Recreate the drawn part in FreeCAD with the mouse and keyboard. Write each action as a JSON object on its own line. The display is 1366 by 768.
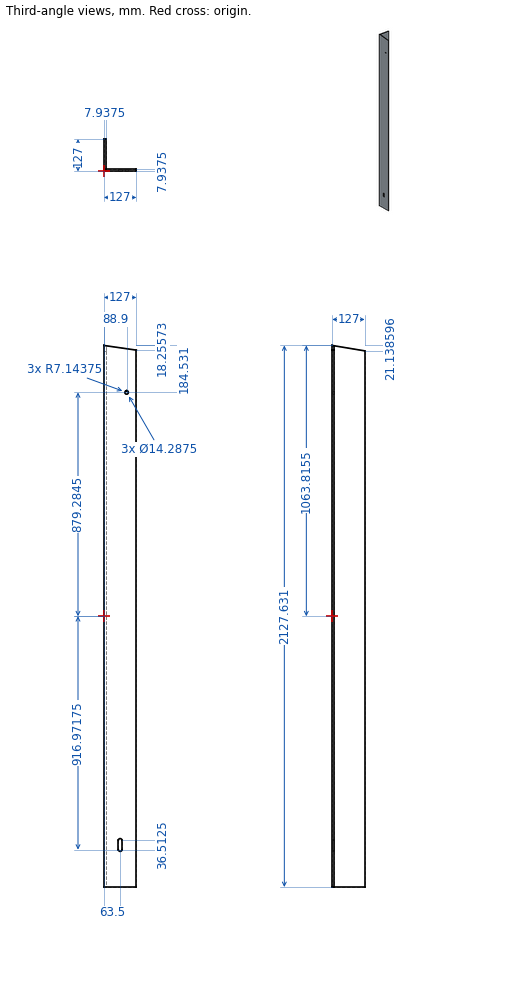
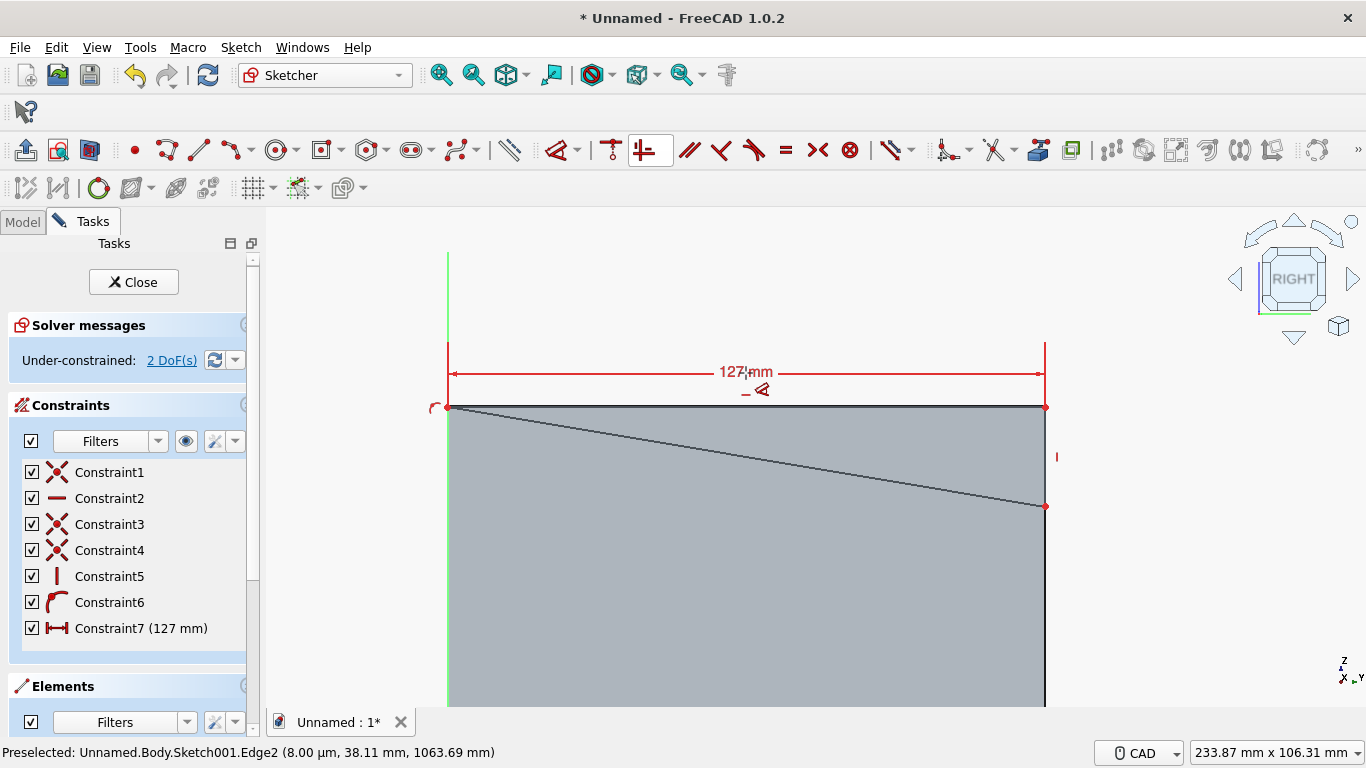
{"action": "left_click", "coordinate": [1045, 437]}
{"action": "left_click", "coordinate": [1079, 457]}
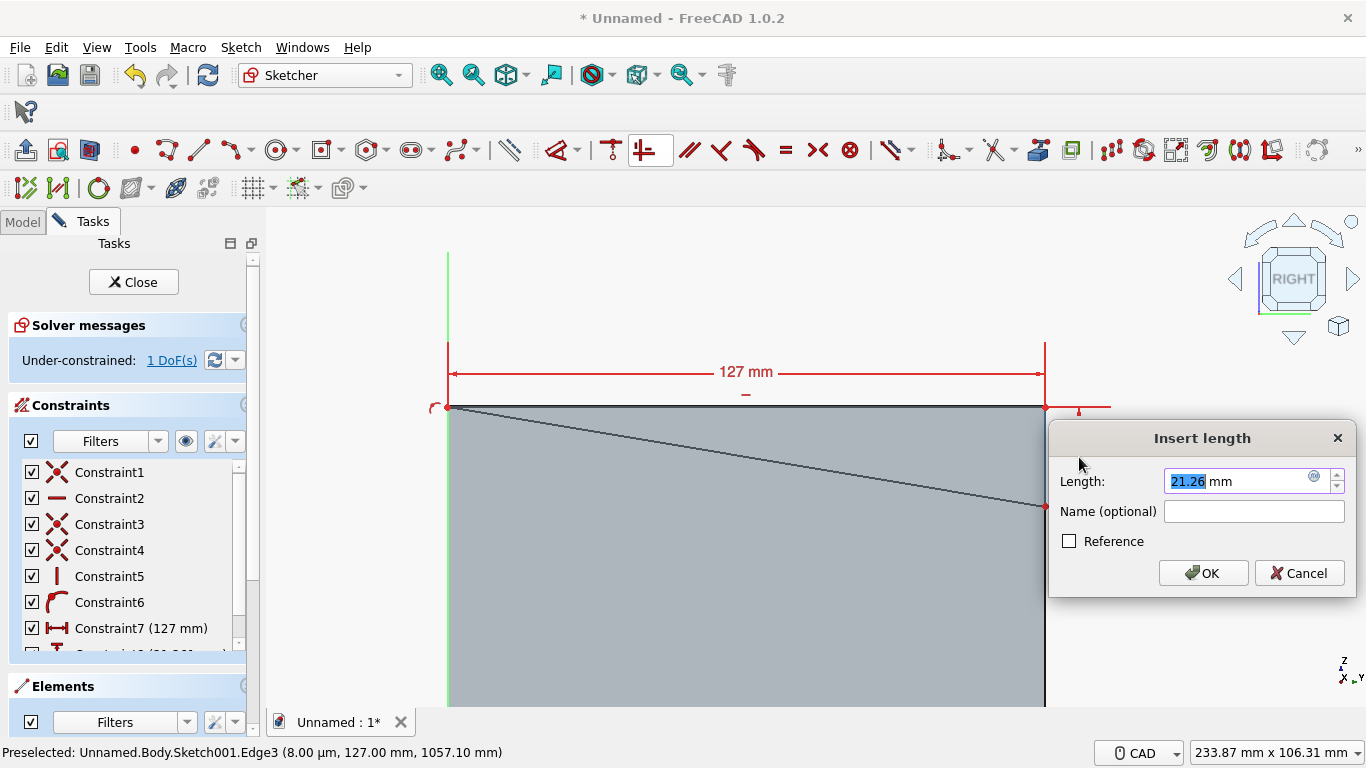
{"action": "type", "text": "21.138596"}
{"action": "key", "text": "Return"}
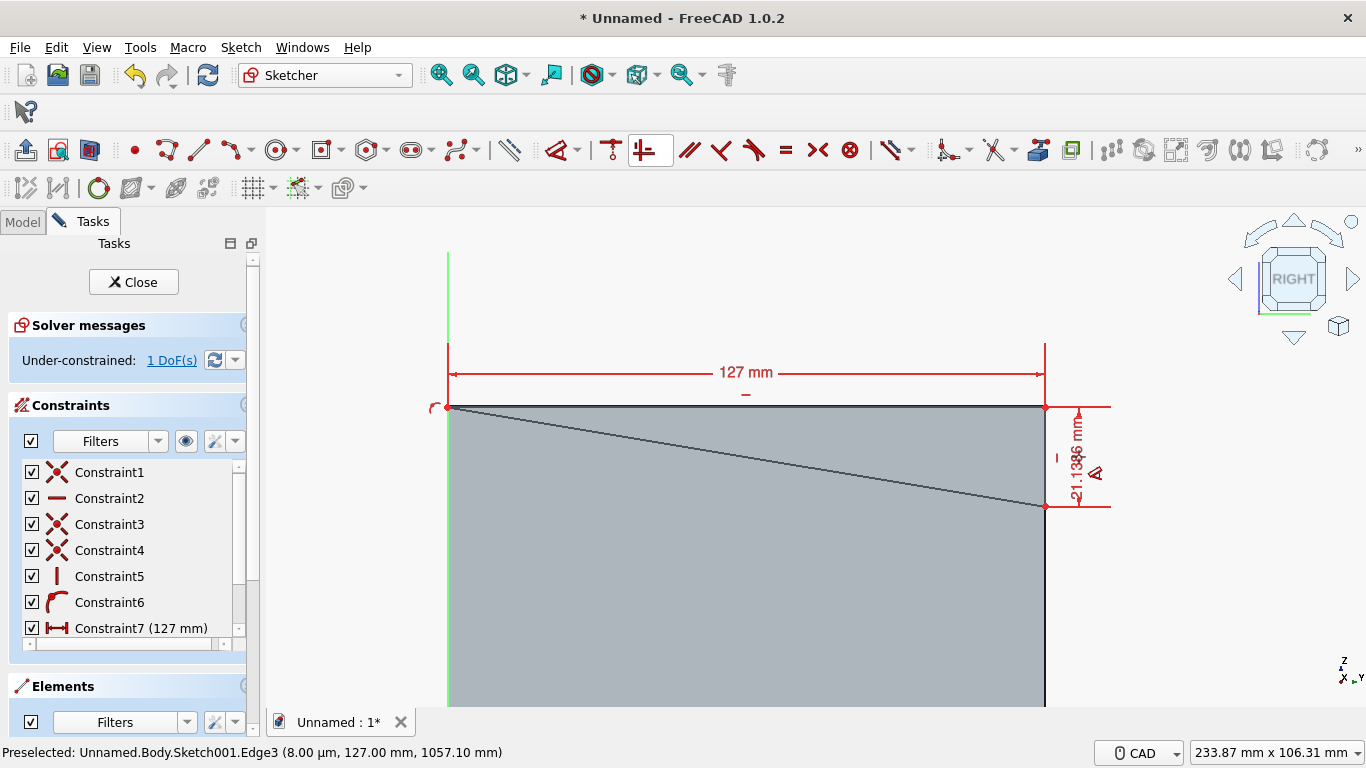
{"action": "left_click", "coordinate": [448, 407]}
{"action": "left_click", "coordinate": [414, 543]}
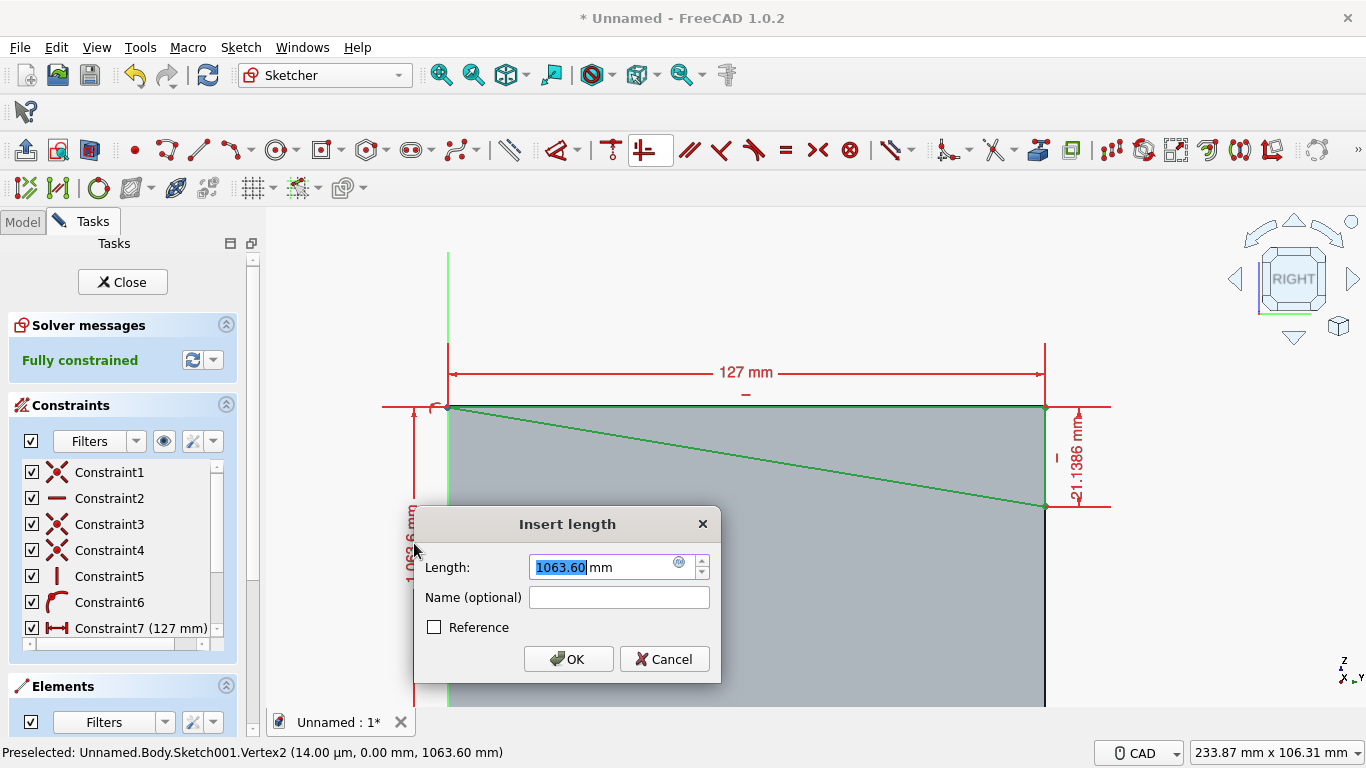
{"action": "type", "text": "1063.8155"}
{"action": "key", "text": "Return"}
{"action": "key", "text": "Escape"}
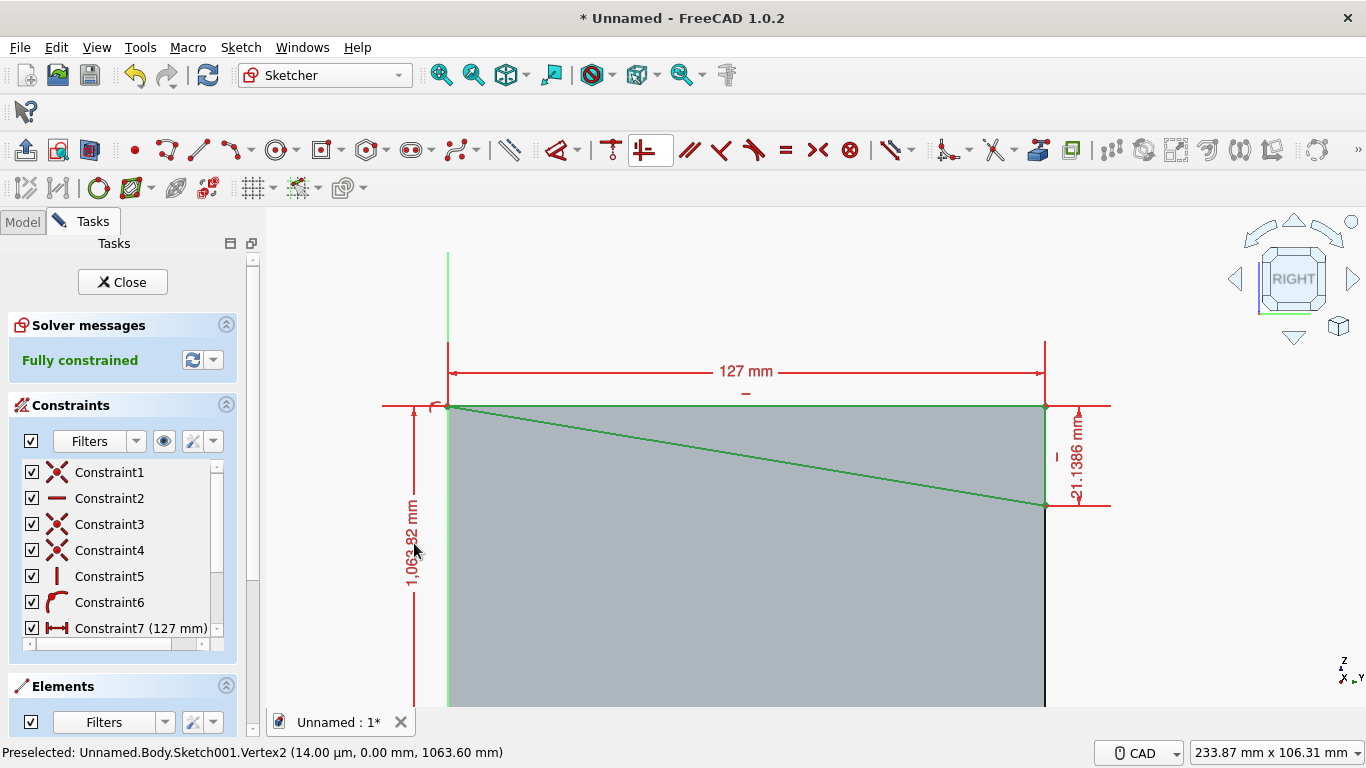
{"action": "left_click", "coordinate": [123, 282]}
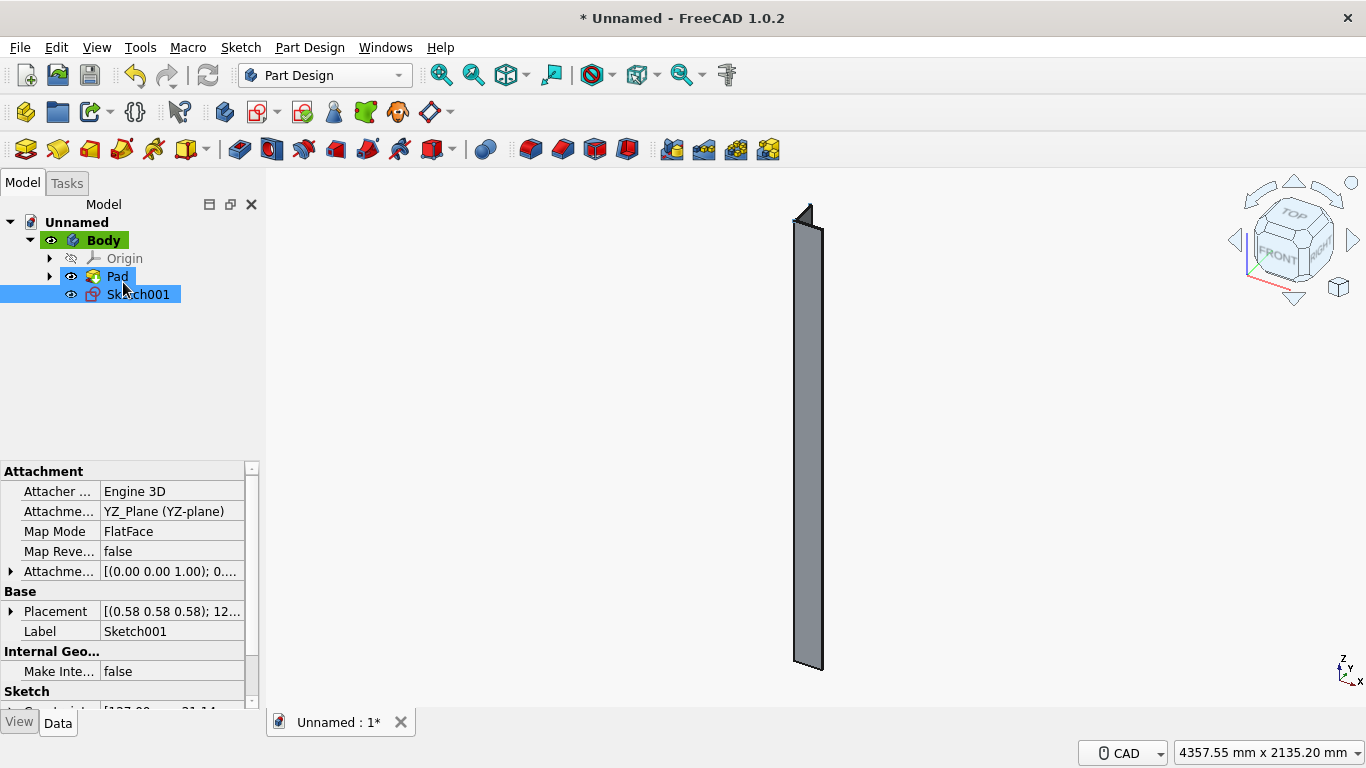
{"action": "left_click", "coordinate": [240, 150]}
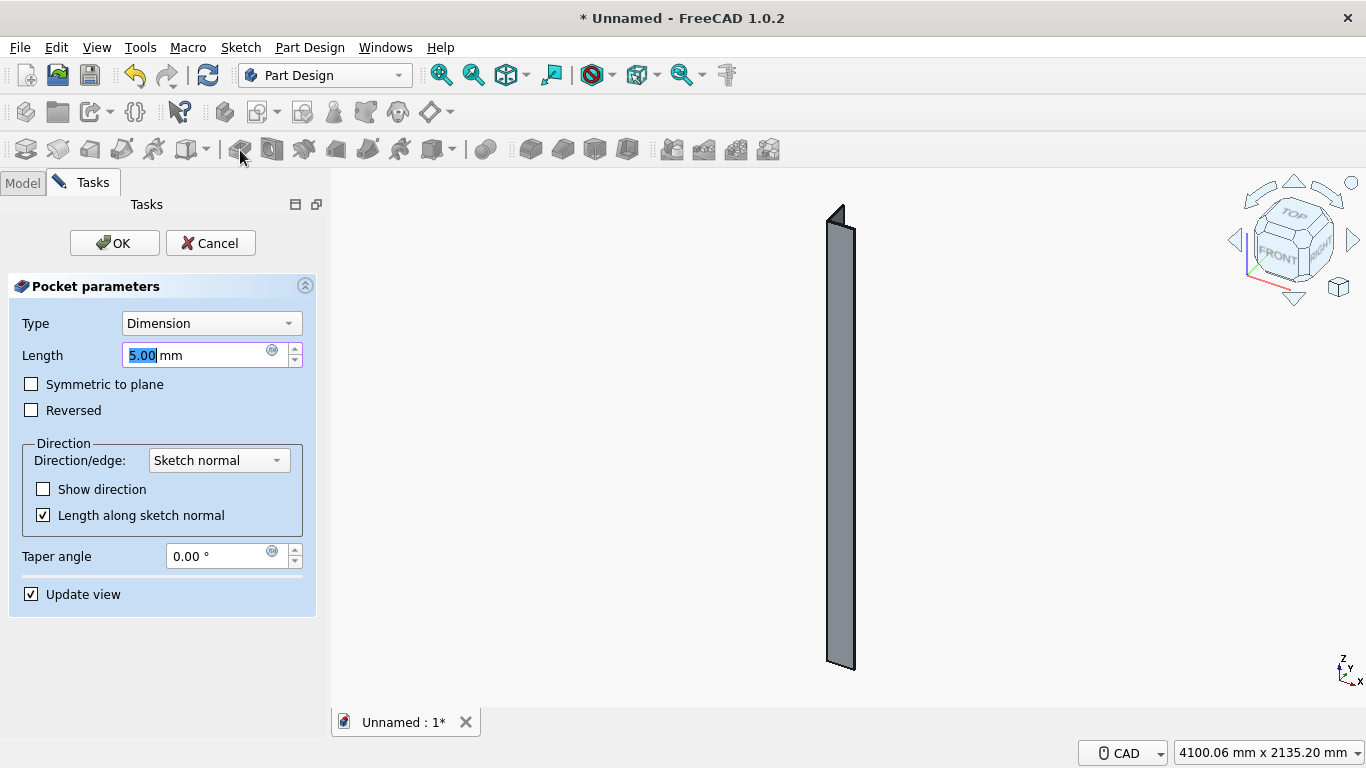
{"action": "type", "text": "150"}
{"action": "key", "text": "Tab"}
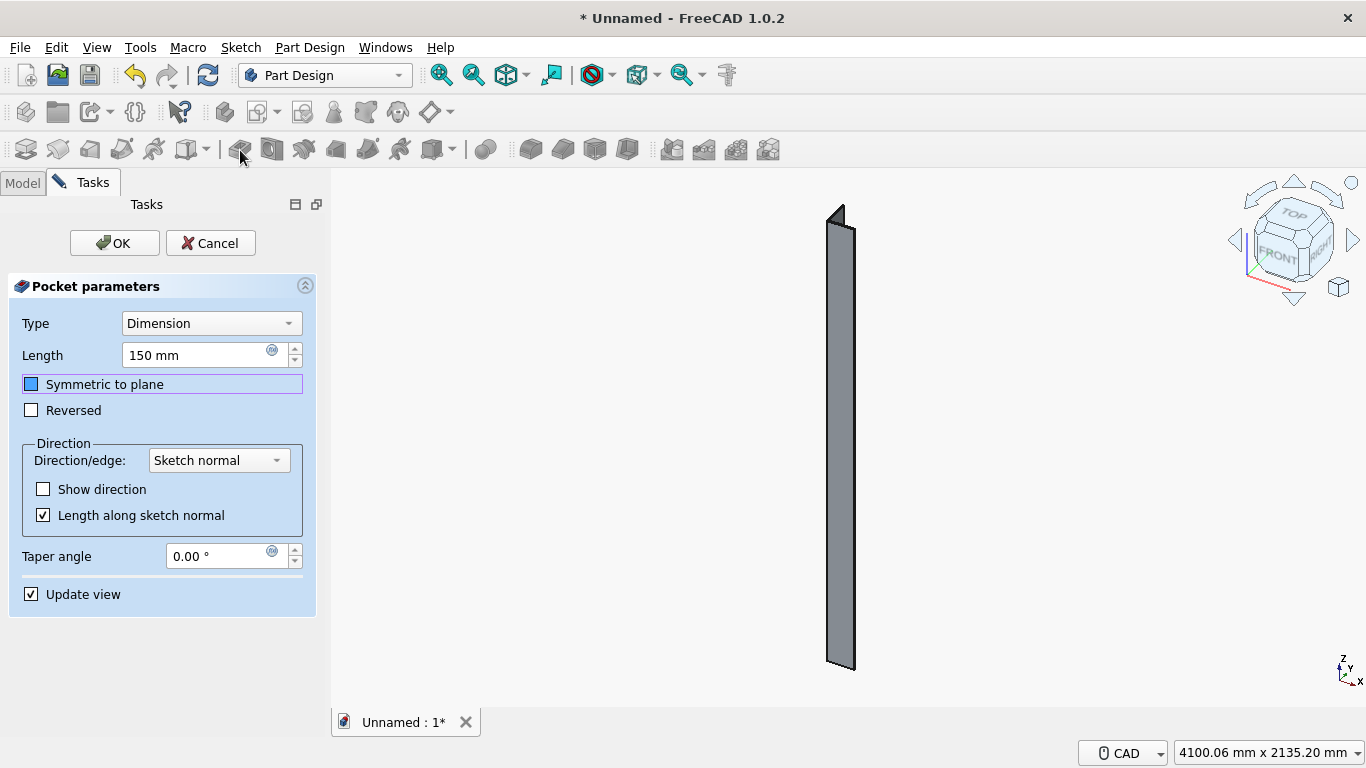
{"action": "left_click", "coordinate": [30, 410]}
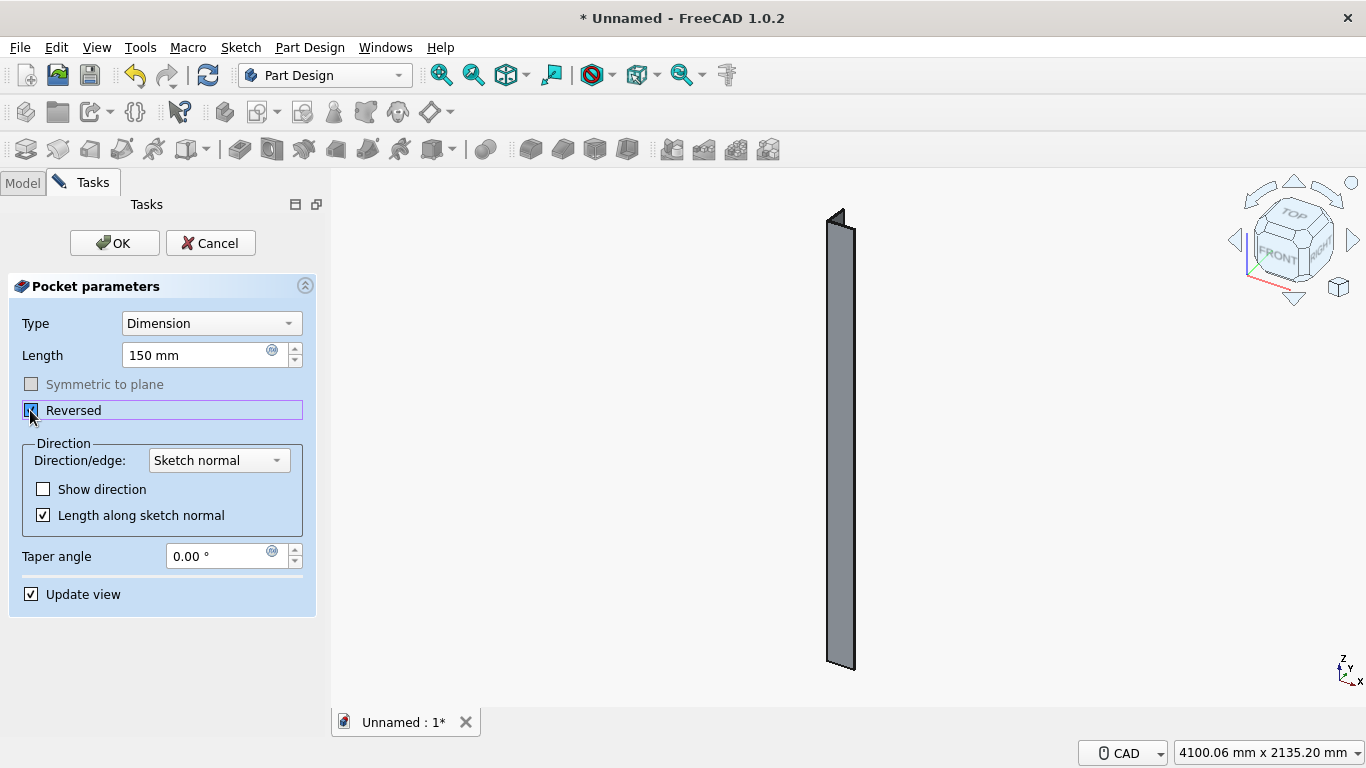
{"action": "left_click", "coordinate": [115, 243]}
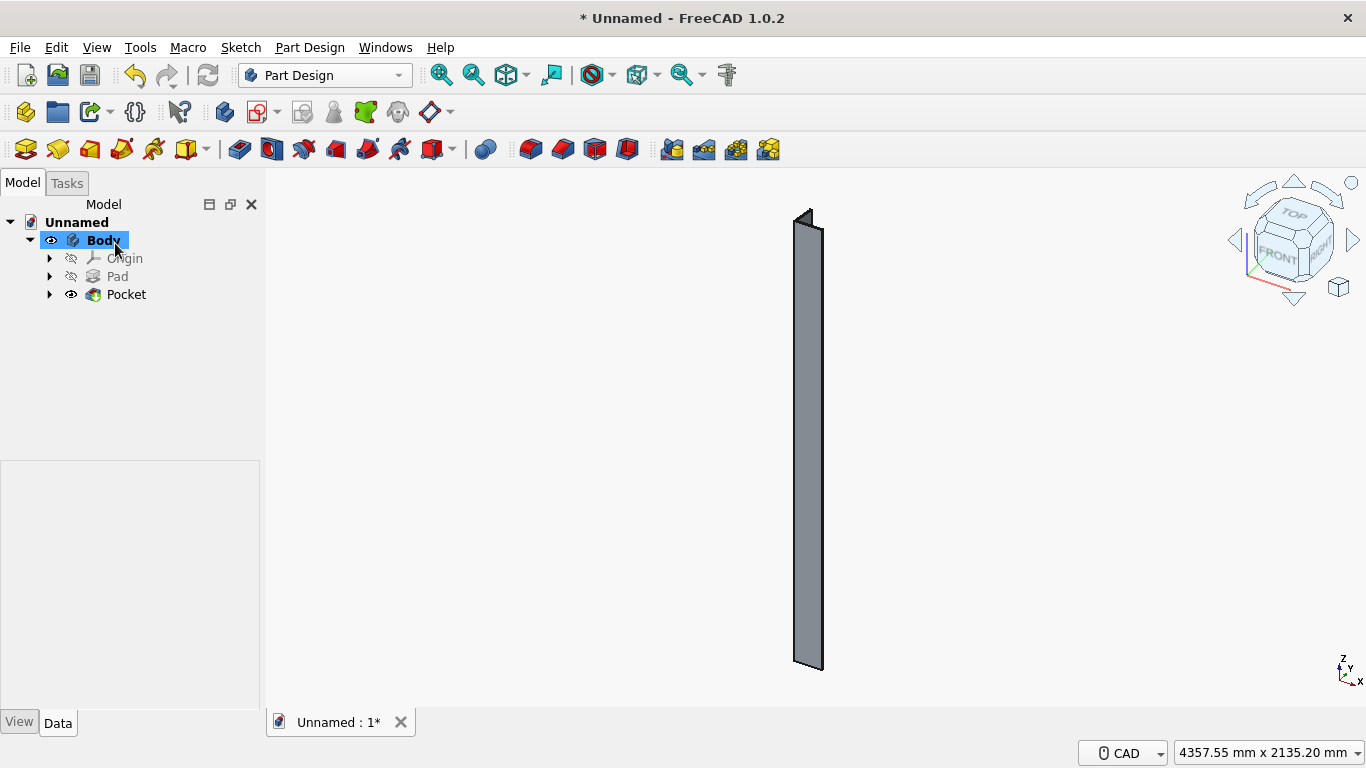
{"action": "key", "text": "4"}